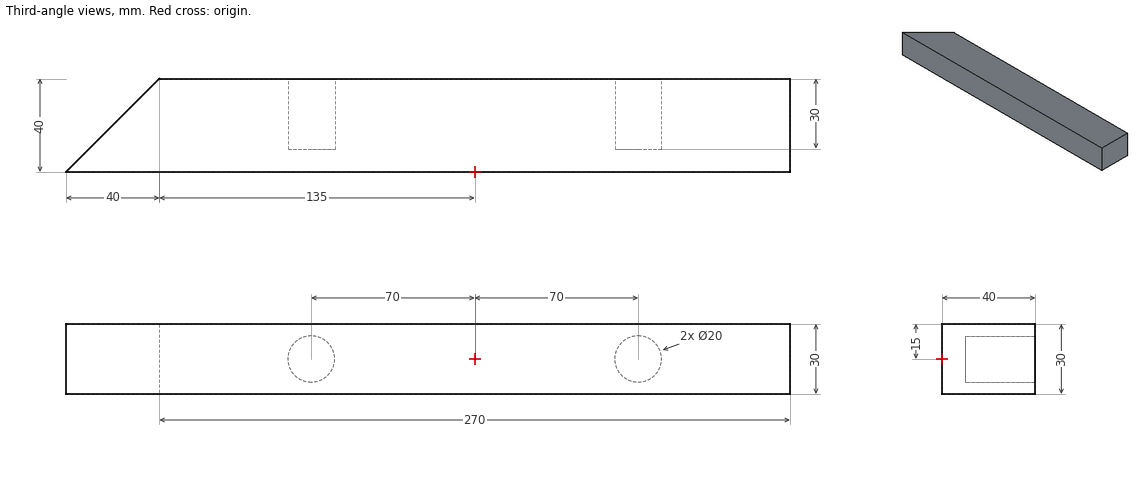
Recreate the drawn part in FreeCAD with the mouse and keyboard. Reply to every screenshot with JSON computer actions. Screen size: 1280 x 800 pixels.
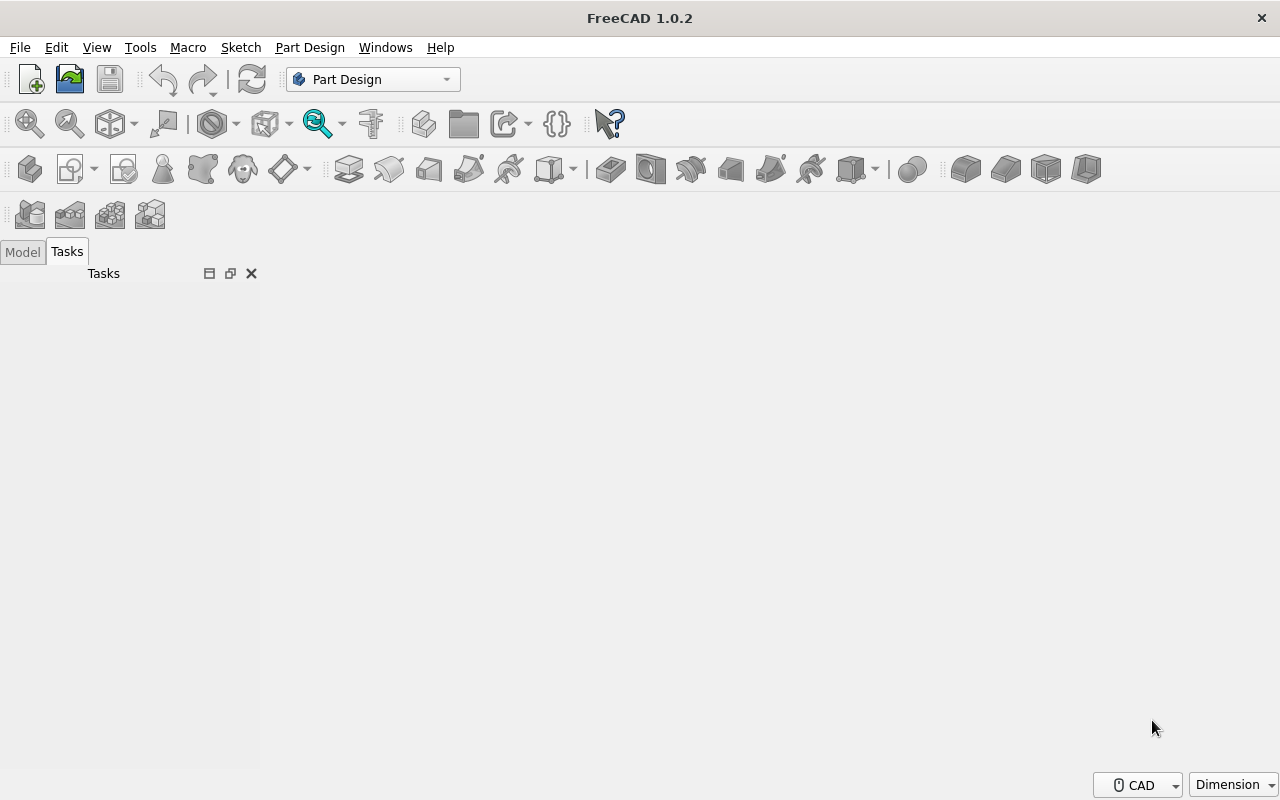
{"action": "left_click", "coordinate": [30, 80]}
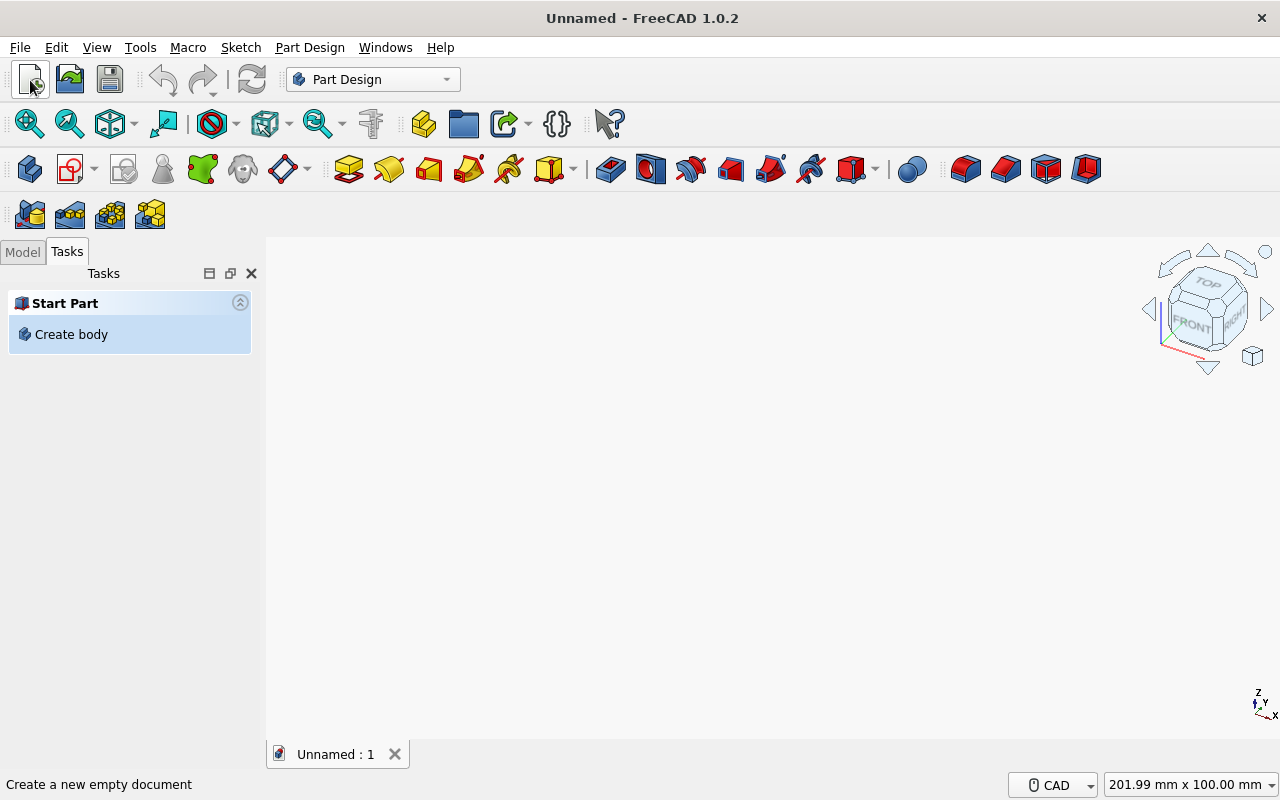
{"action": "left_click", "coordinate": [70, 170]}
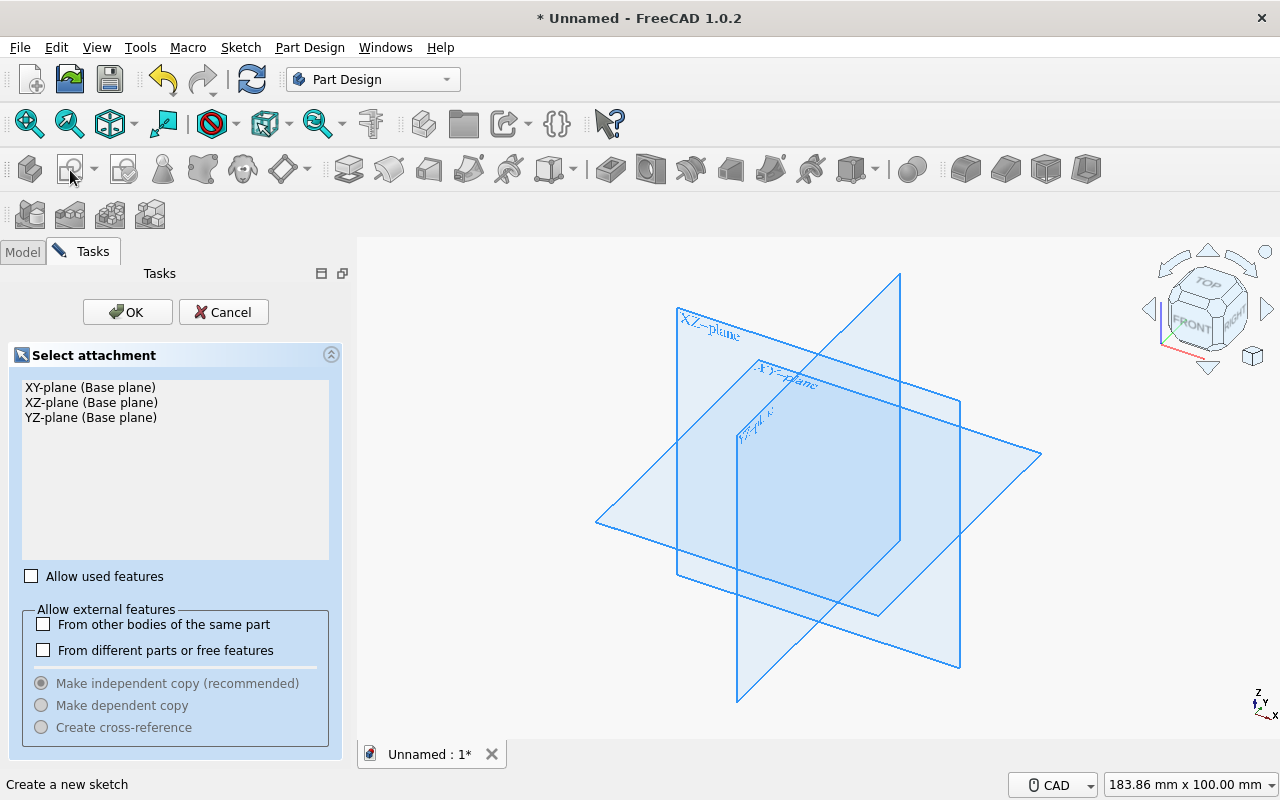
{"action": "left_click", "coordinate": [82, 402]}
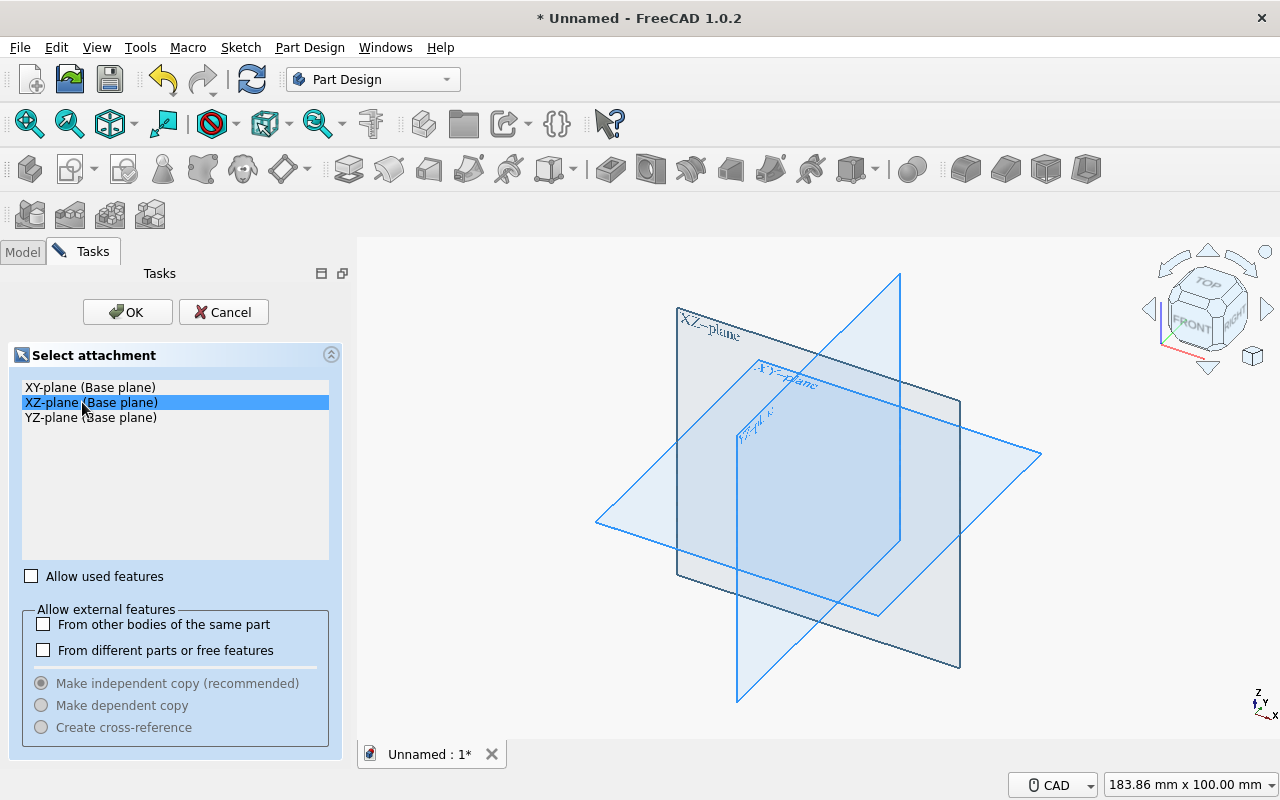
{"action": "left_click", "coordinate": [128, 312]}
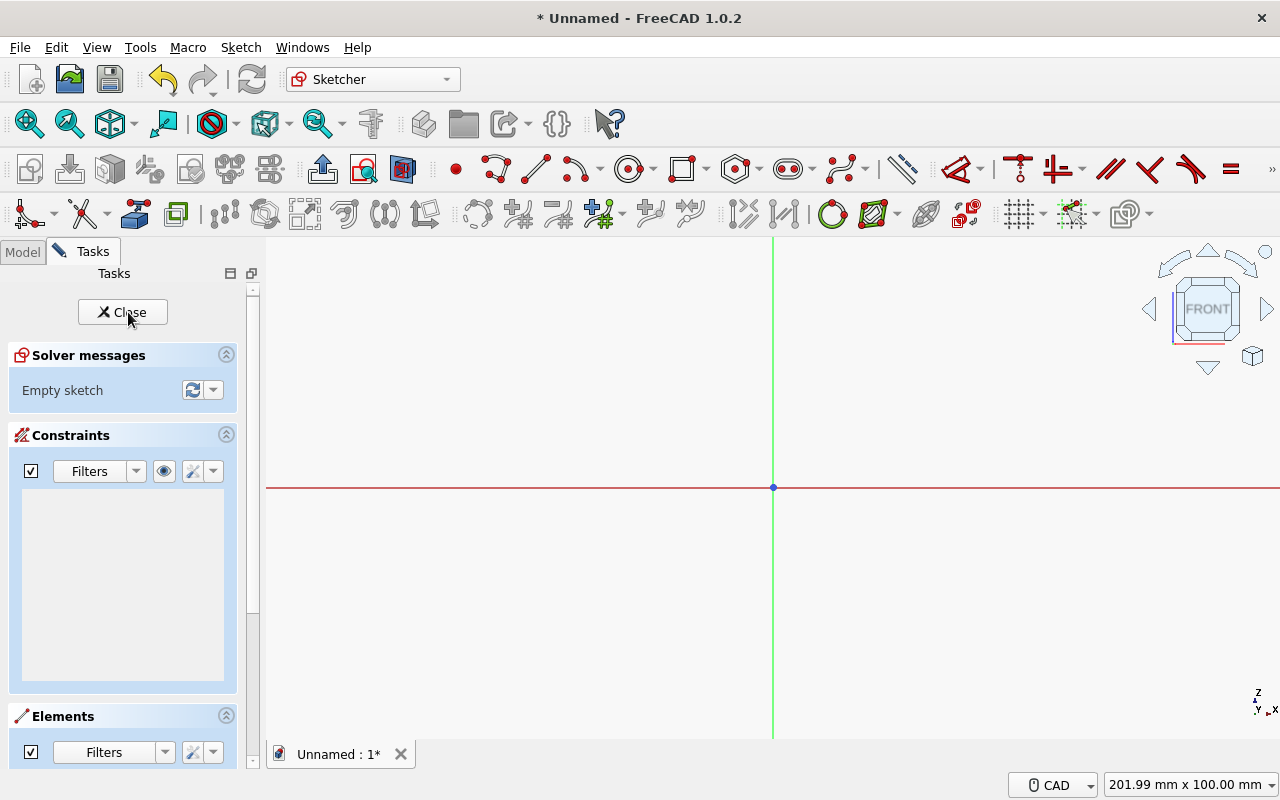
{"action": "scroll", "coordinate": [649, 488], "scroll_direction": "down", "scroll_amount": 4}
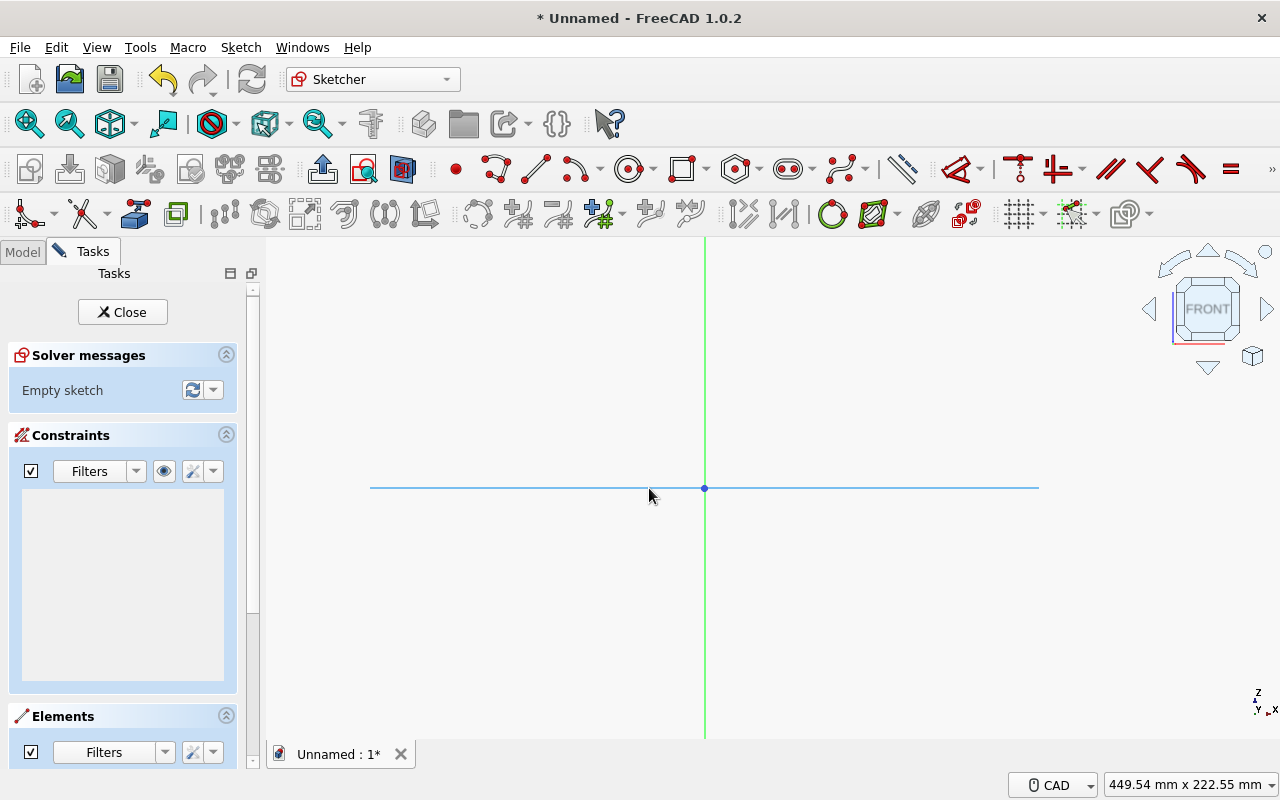
{"action": "left_click", "coordinate": [708, 170]}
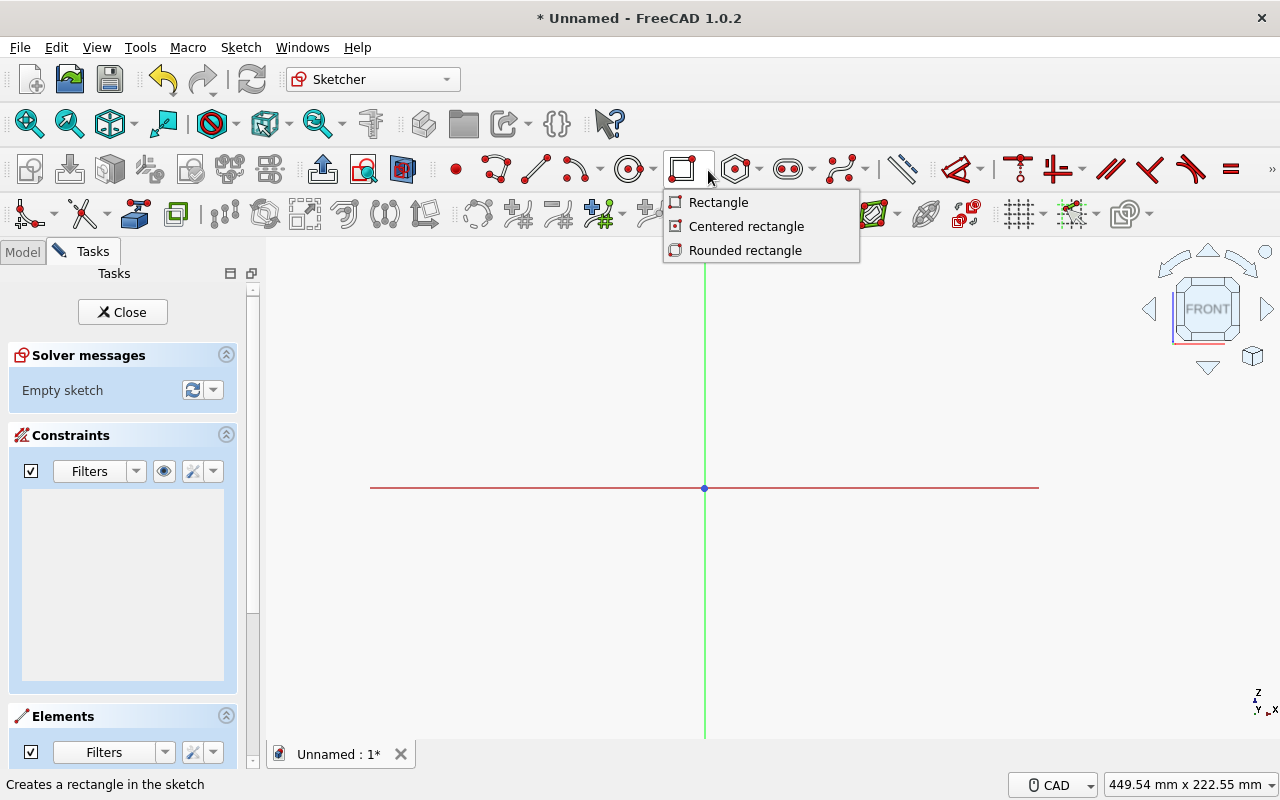
{"action": "left_click", "coordinate": [762, 226]}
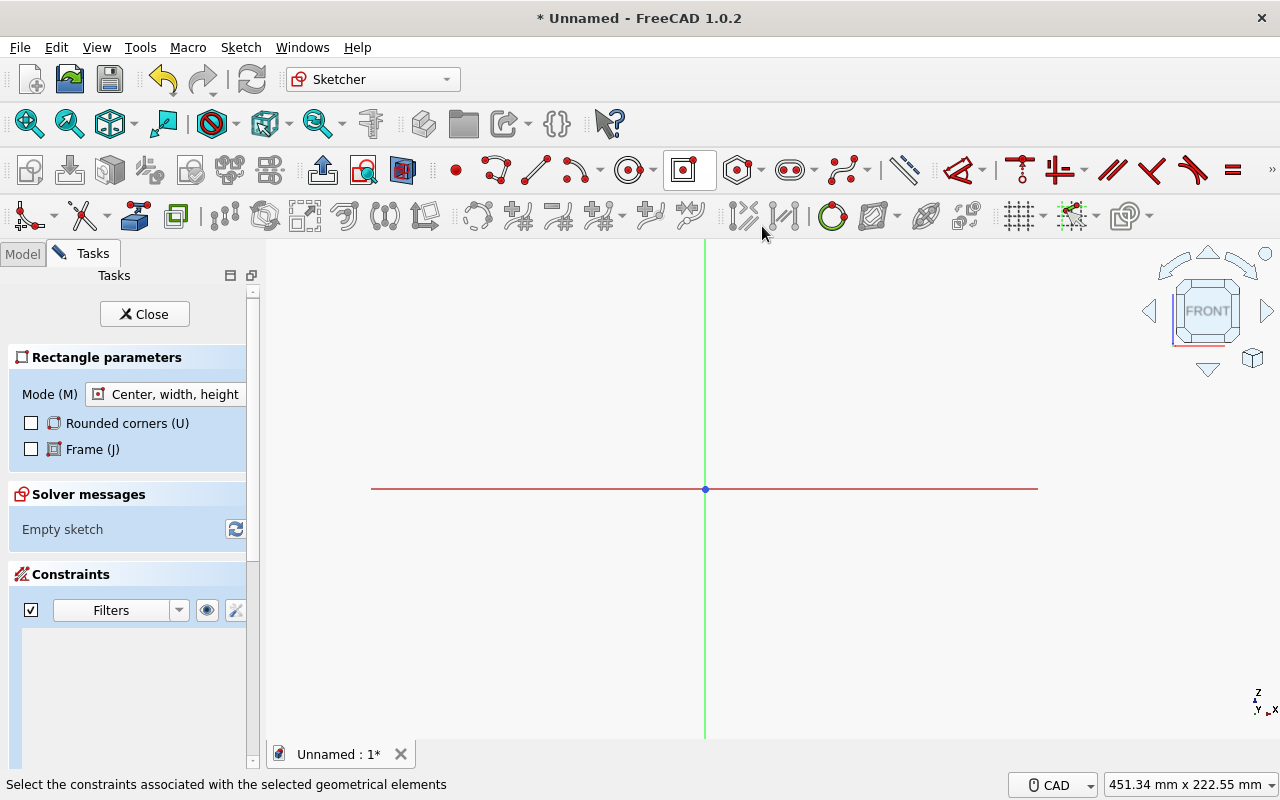
{"action": "left_click", "coordinate": [705, 489]}
{"action": "mouse_move", "coordinate": [1008, 456]}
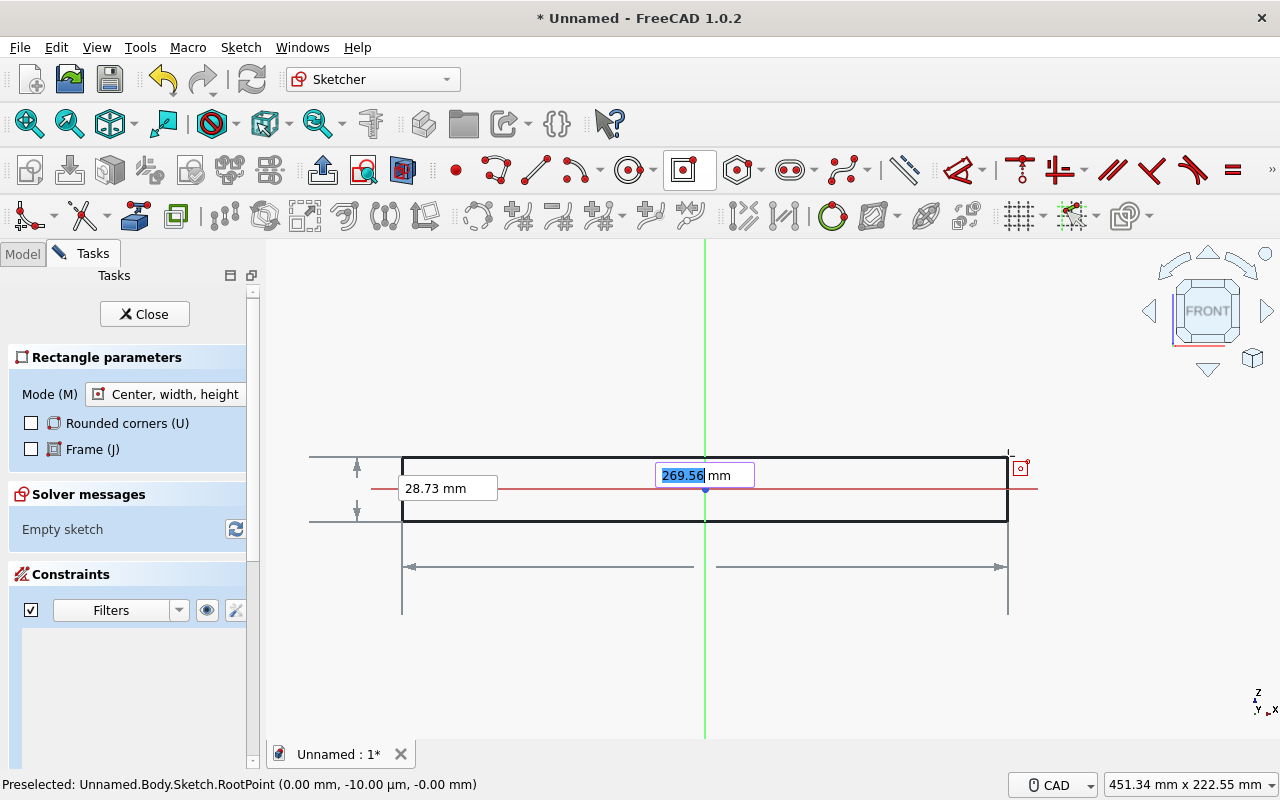
{"action": "type", "text": "270"}
{"action": "key", "text": "Tab"}
{"action": "type", "text": "30"}
{"action": "key", "text": "Return"}
{"action": "key", "text": "Escape"}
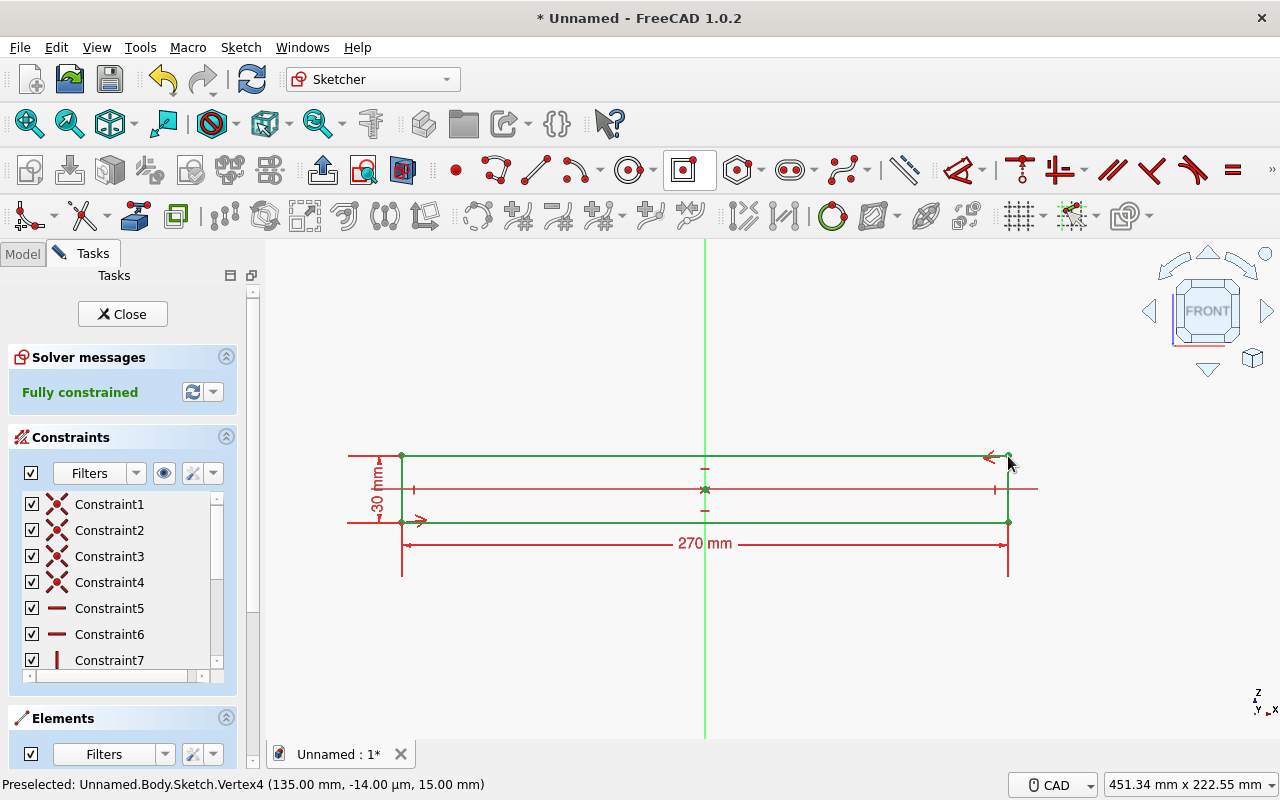
{"action": "left_click", "coordinate": [123, 314]}